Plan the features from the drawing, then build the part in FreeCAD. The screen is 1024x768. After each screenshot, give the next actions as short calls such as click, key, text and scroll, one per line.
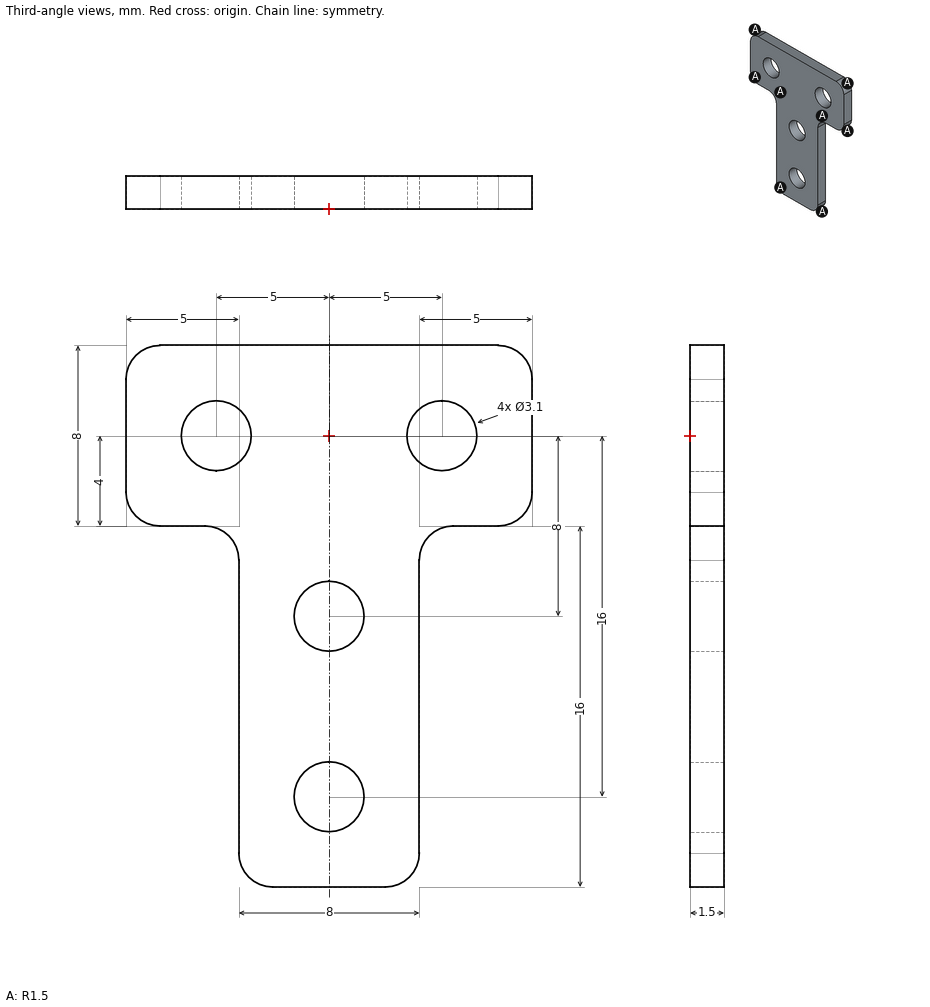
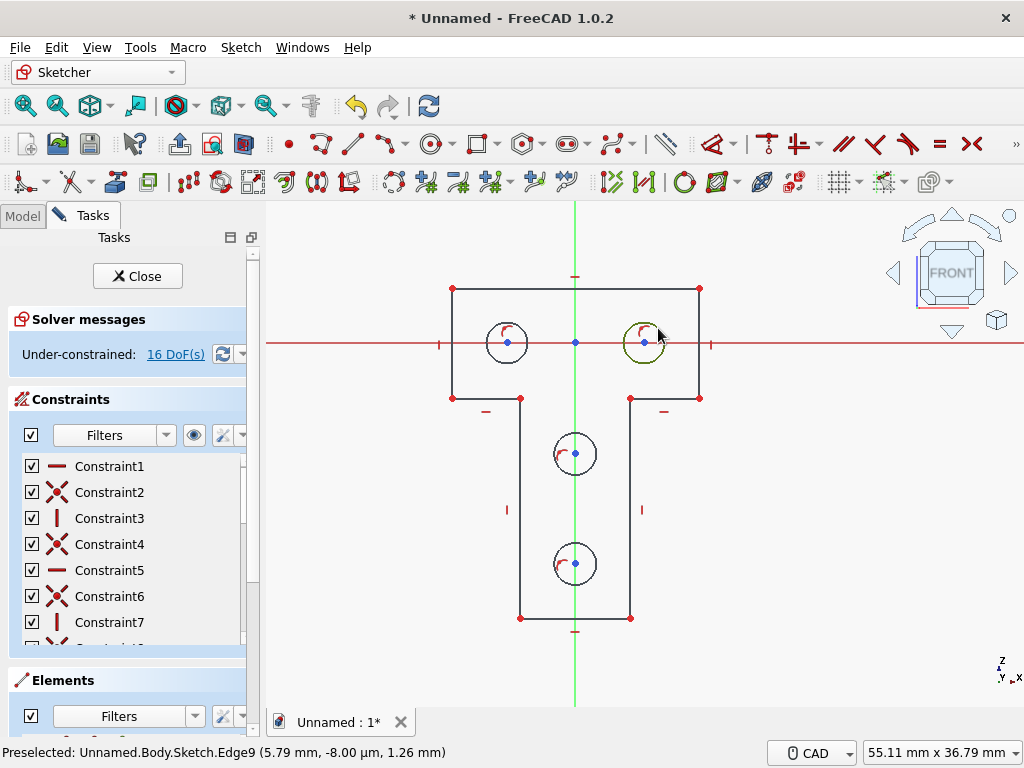
click(521, 328)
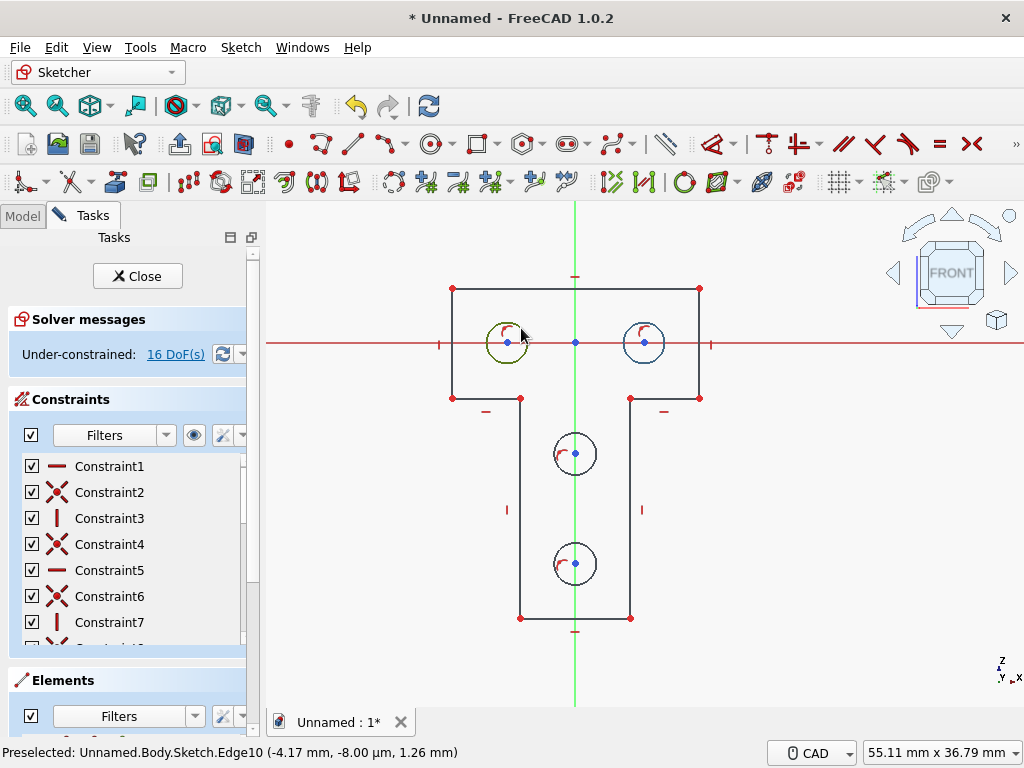
click(590, 439)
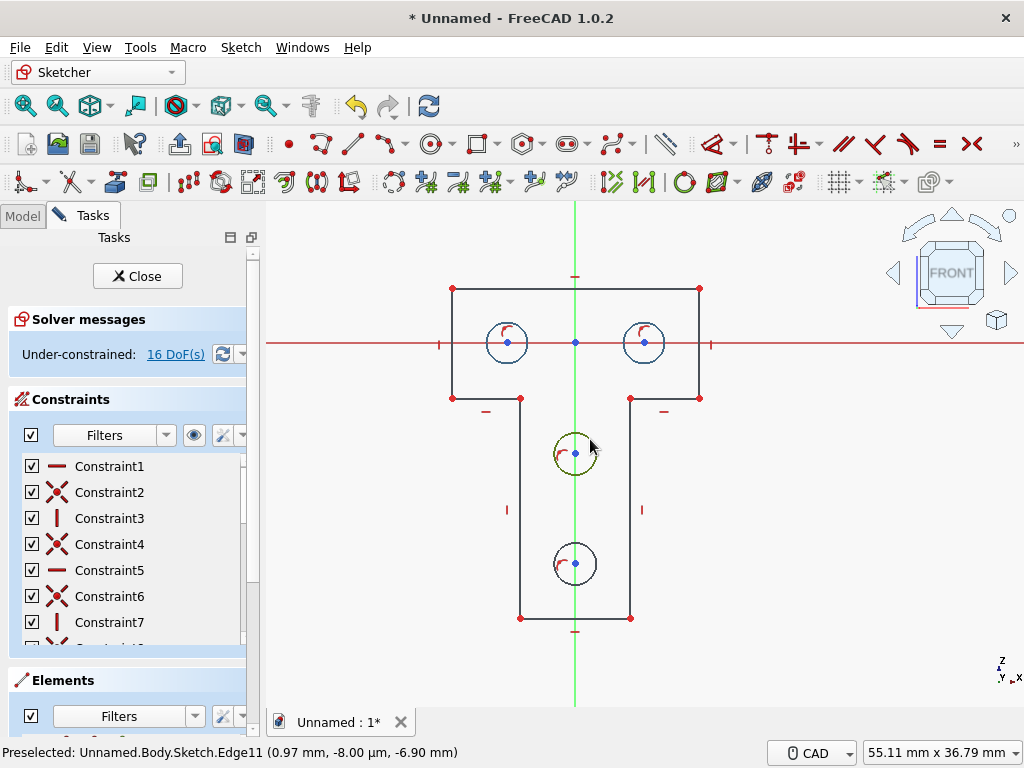
click(590, 549)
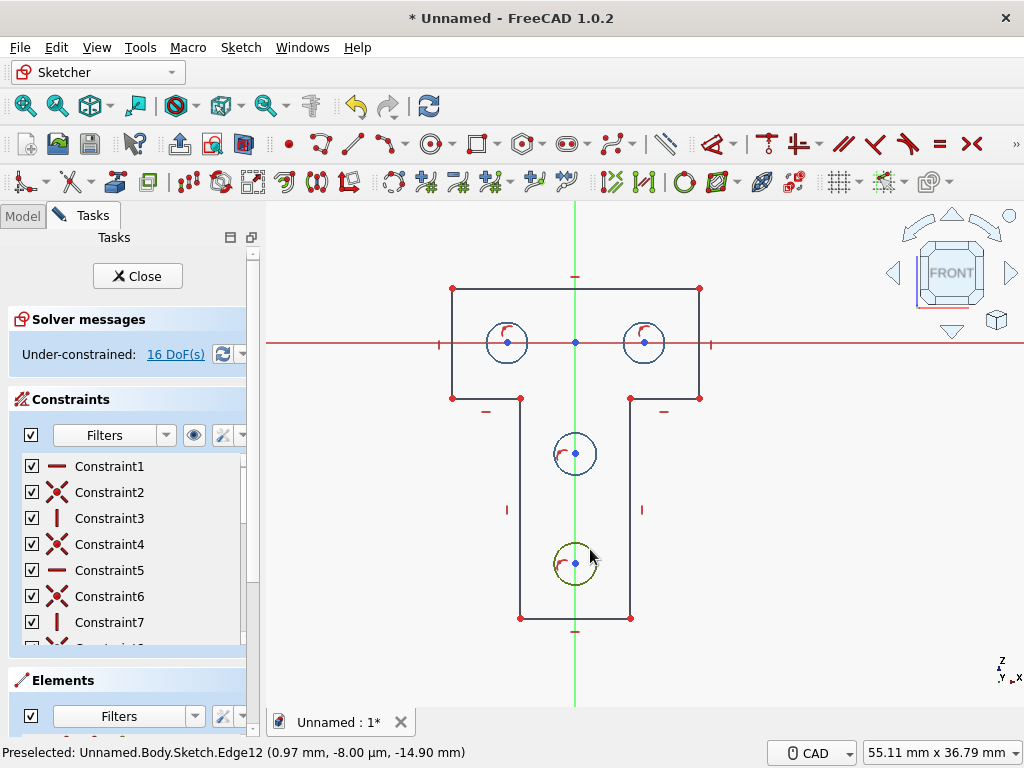
click(940, 144)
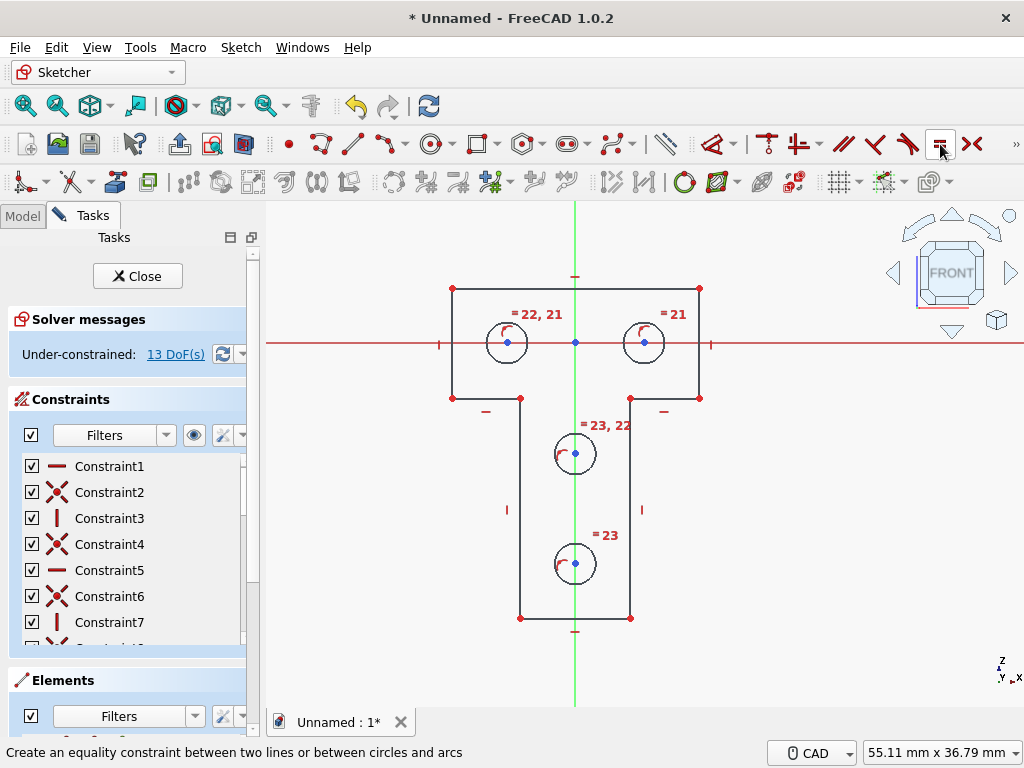
click(452, 399)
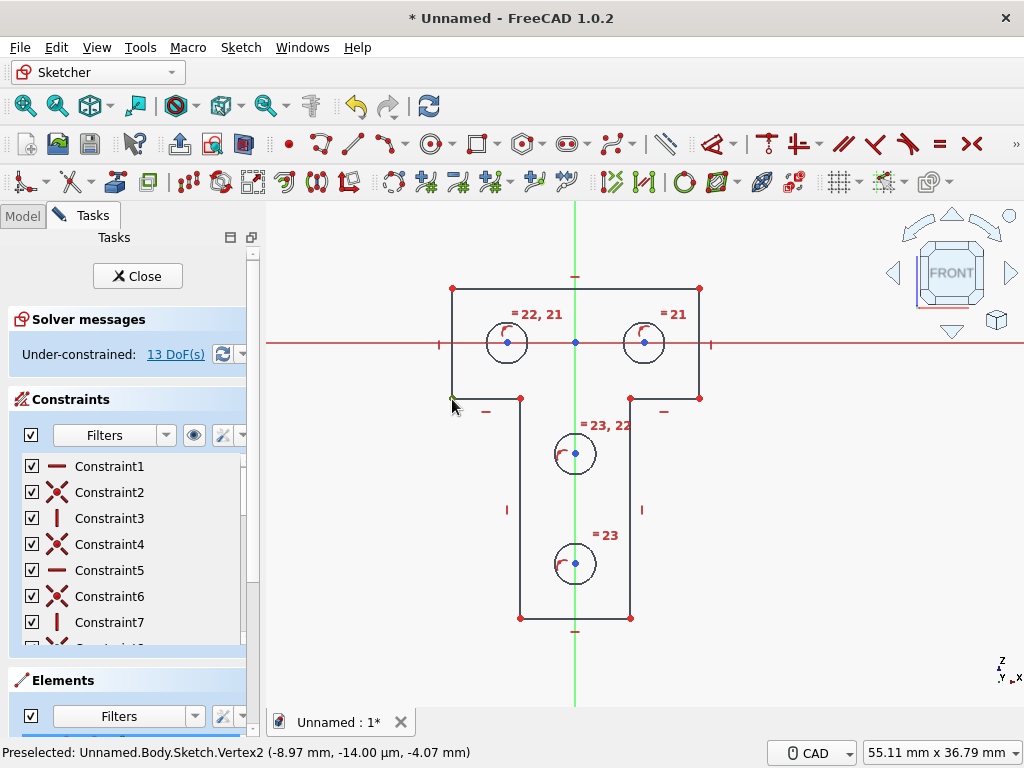
click(699, 399)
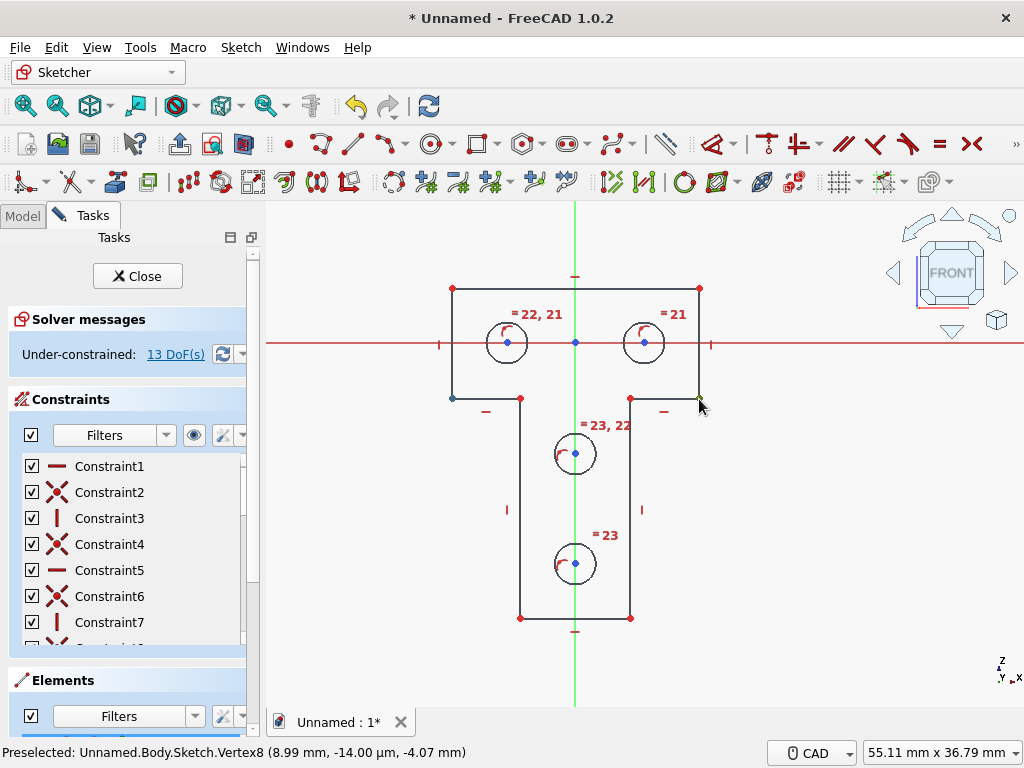
click(575, 390)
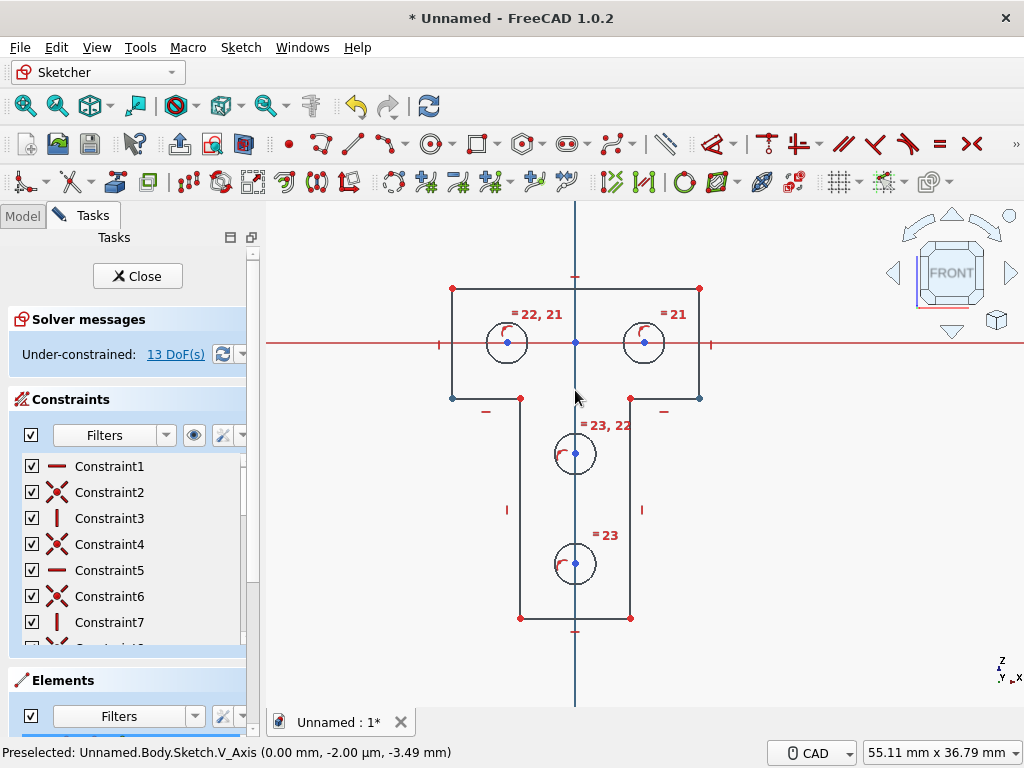
click(972, 144)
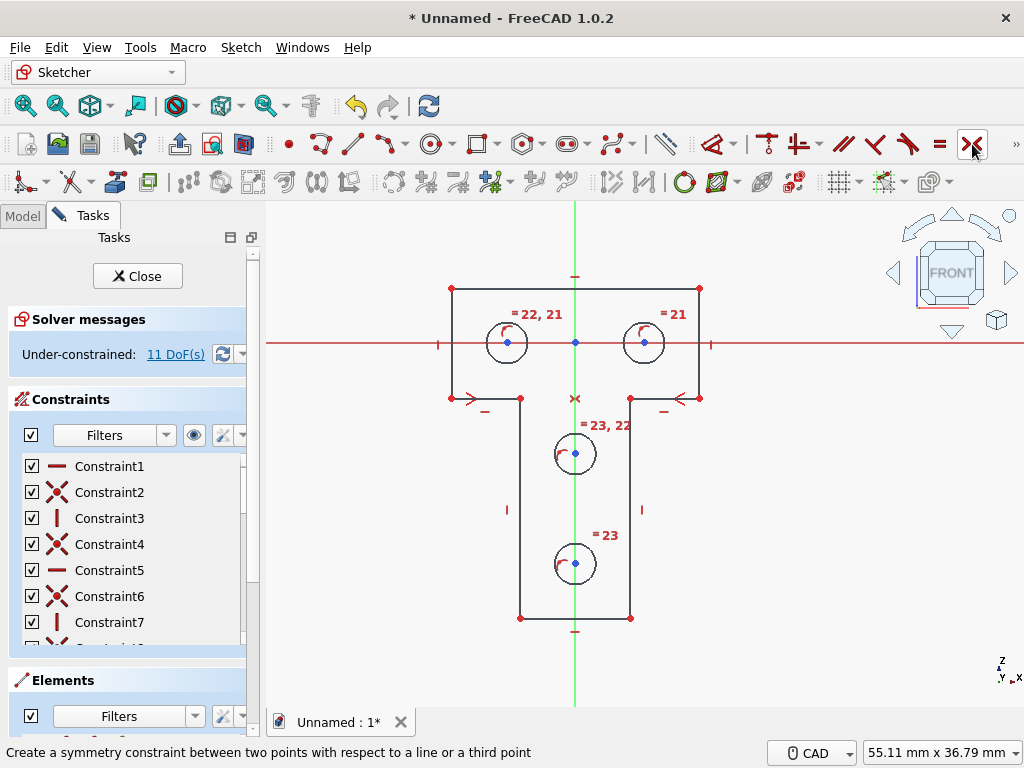
click(712, 144)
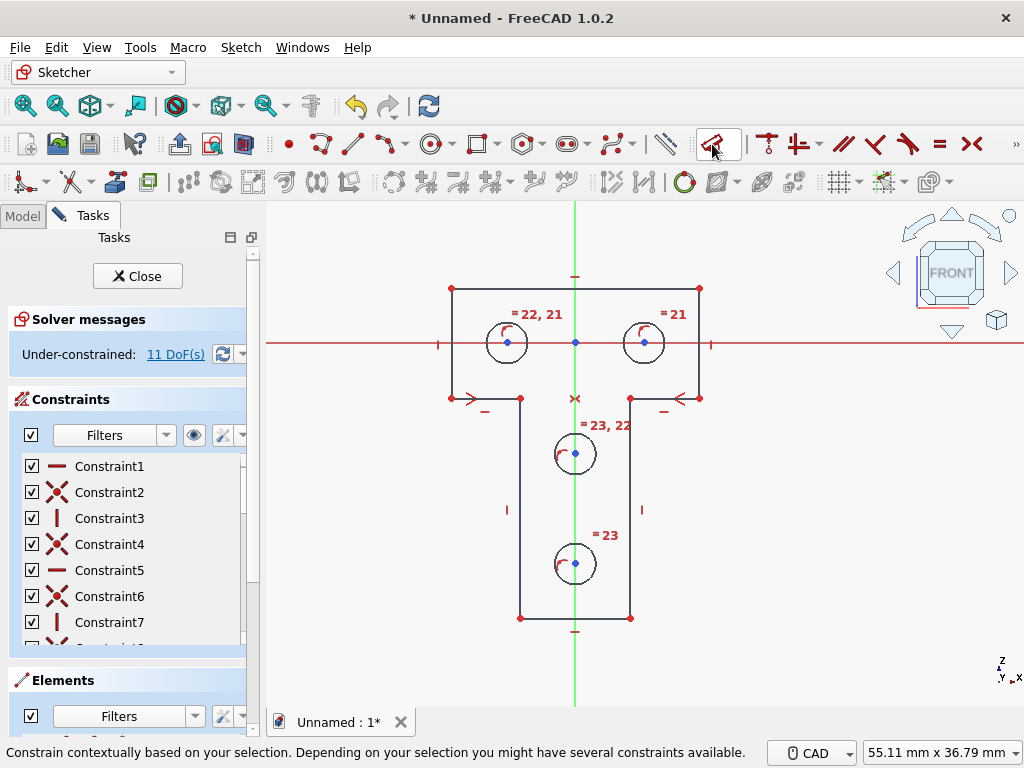
click(658, 328)
click(680, 305)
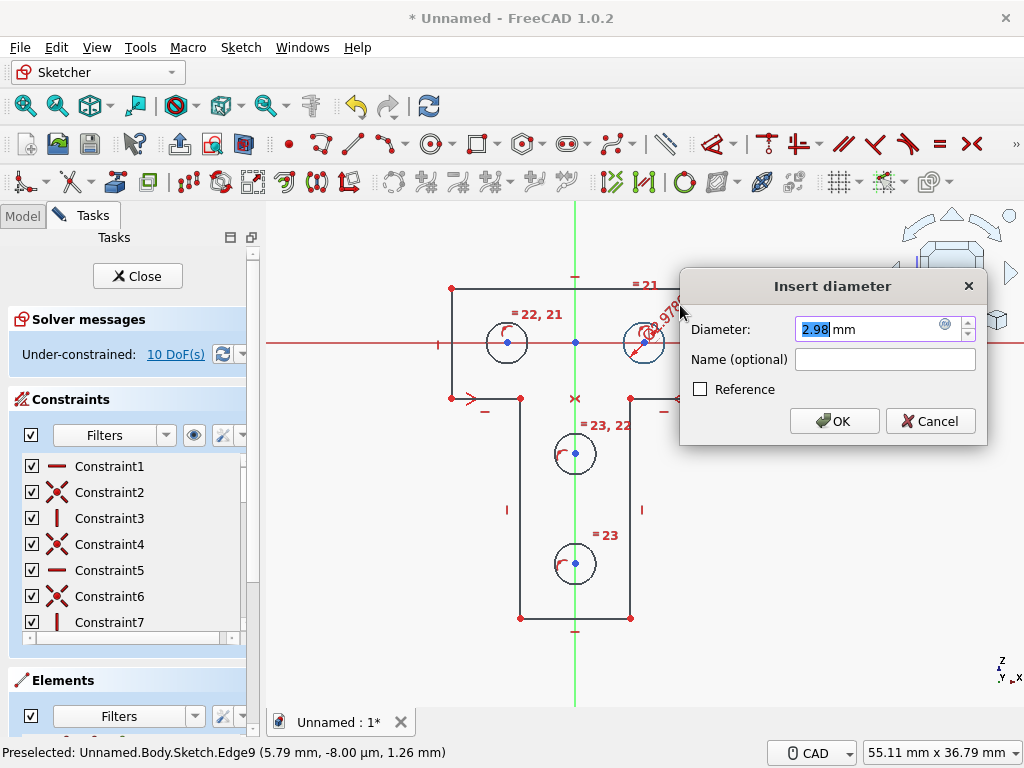
text(3.1)
key(Return)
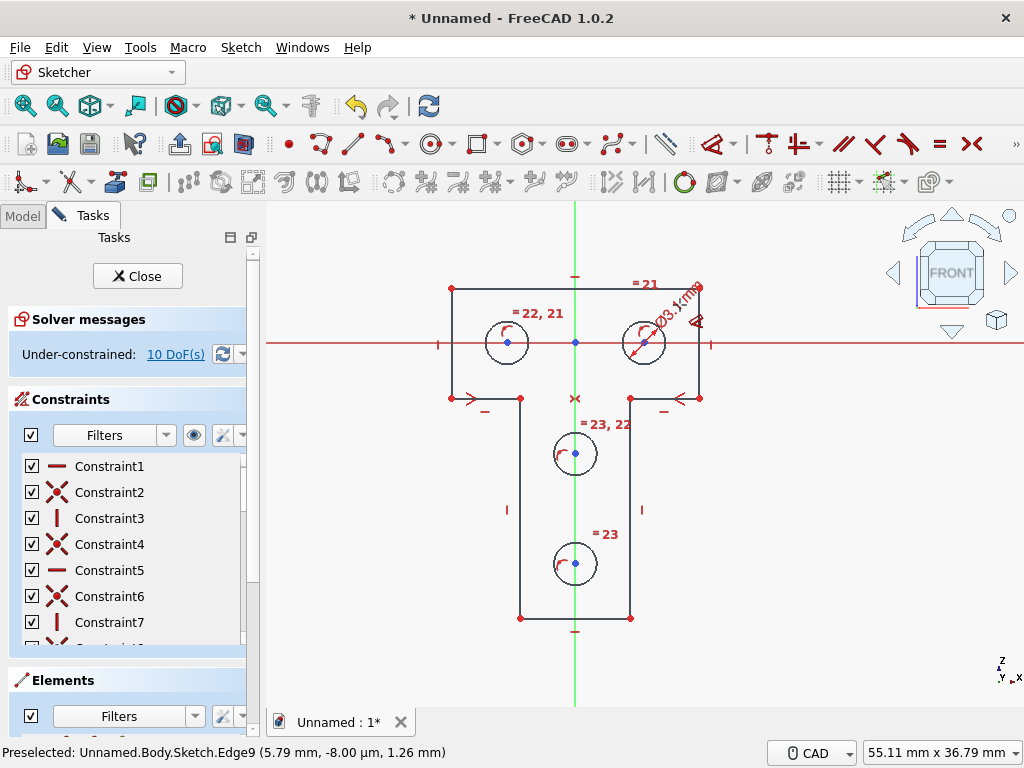
click(499, 399)
click(470, 365)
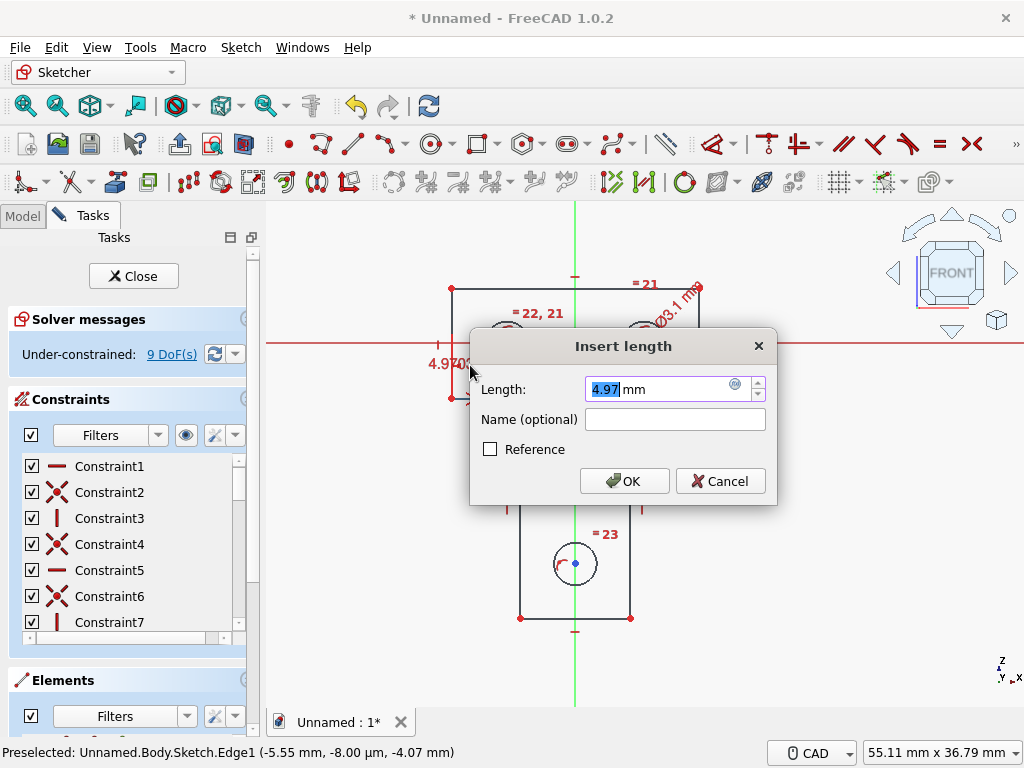
text(5)
key(Return)